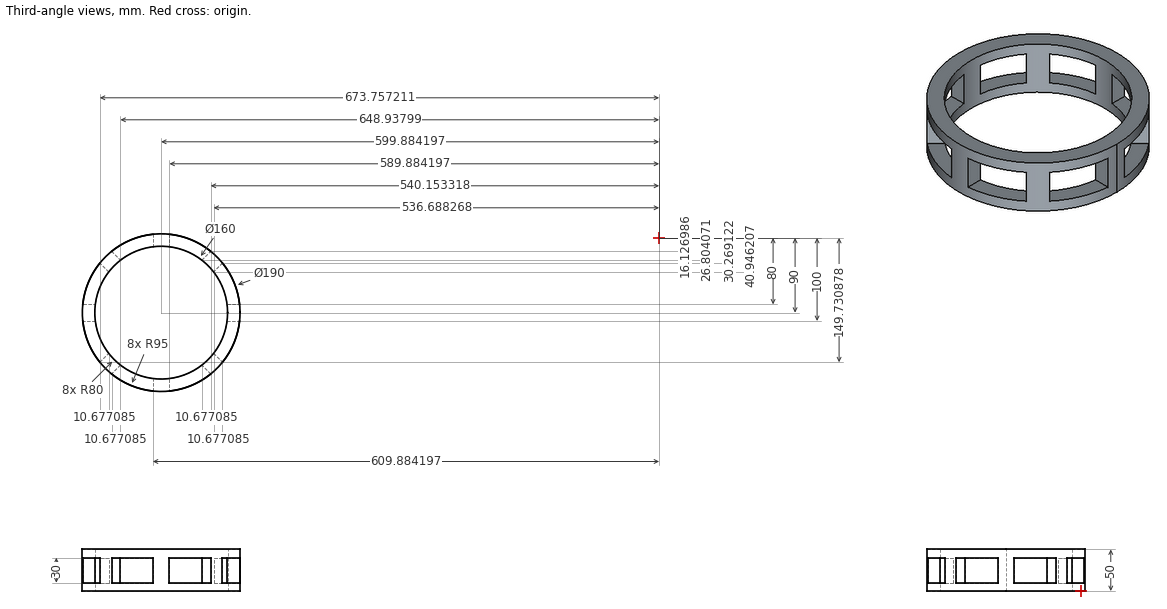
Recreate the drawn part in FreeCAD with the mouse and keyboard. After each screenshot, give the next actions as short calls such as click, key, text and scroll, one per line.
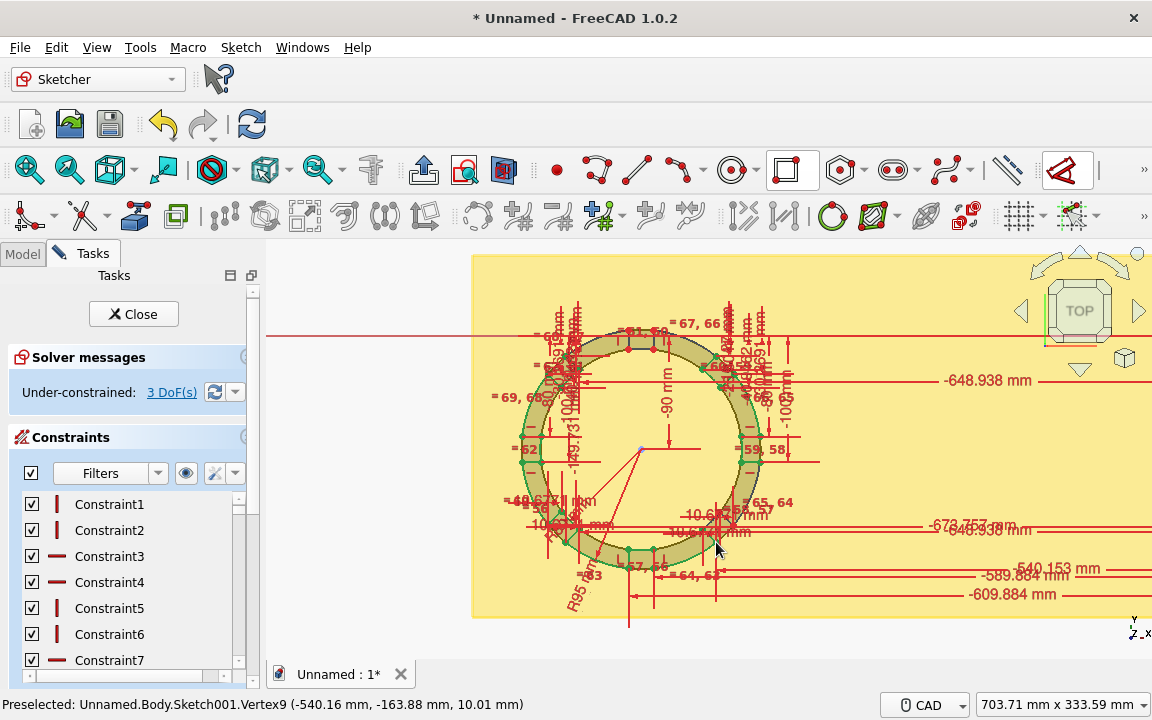
click(720, 512)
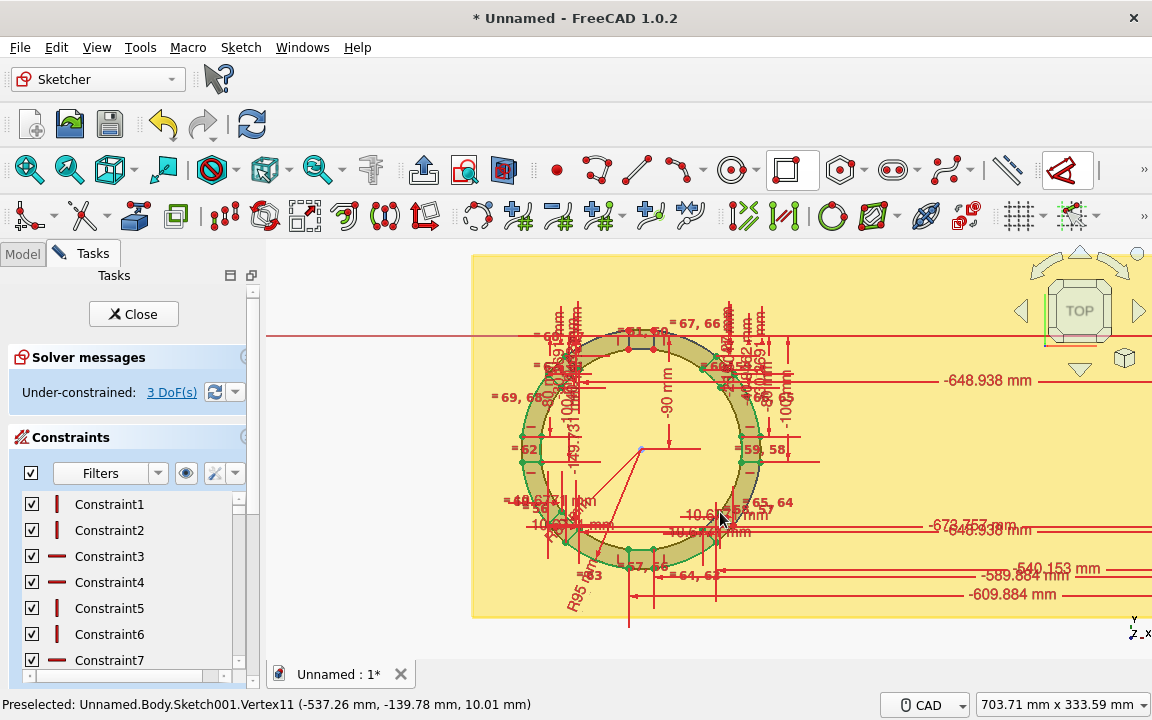
key(l)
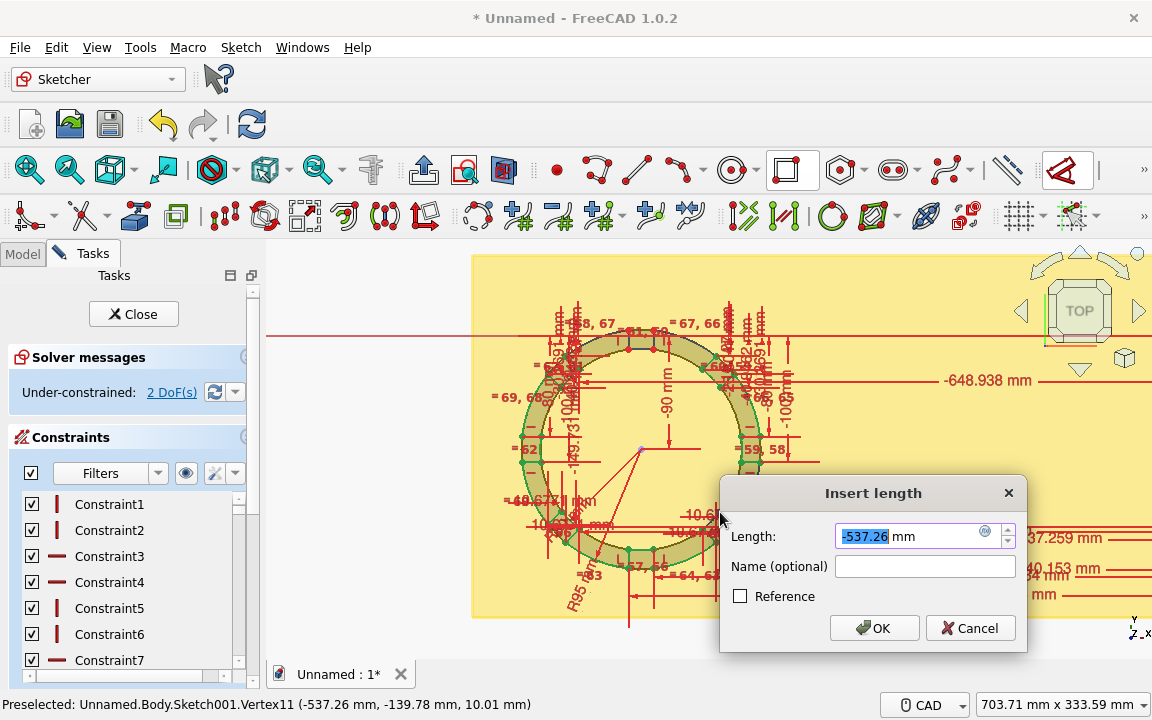
text(-536.688268)
key(Return)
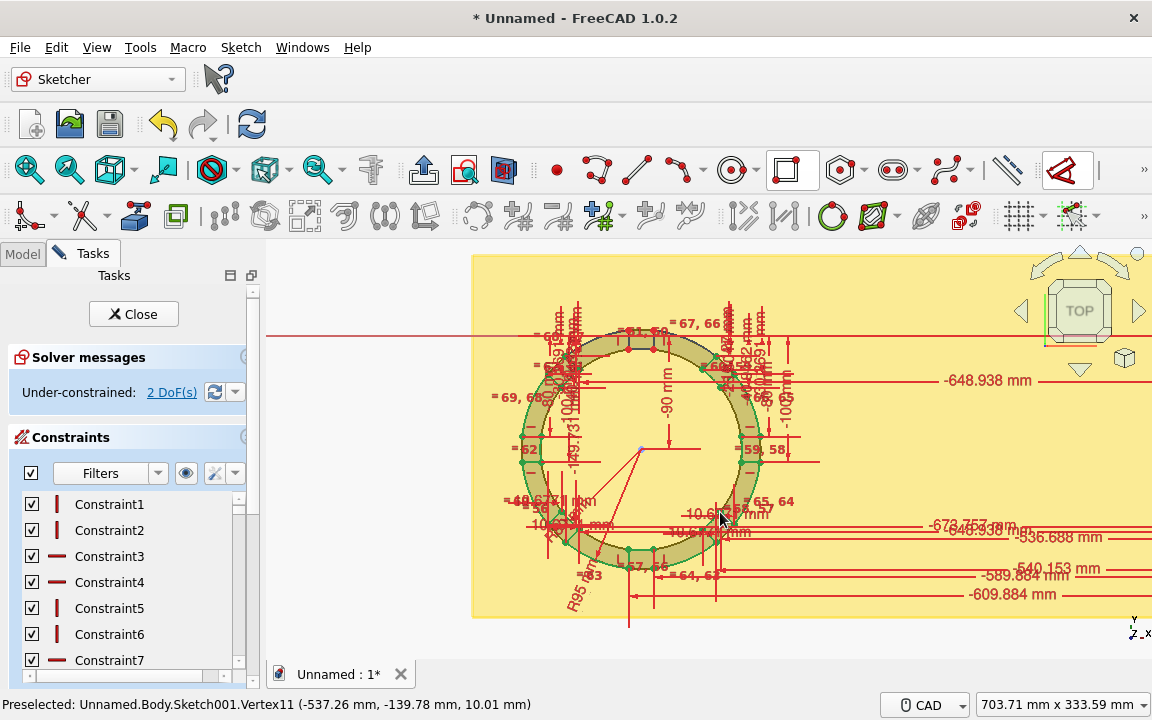
click(654, 331)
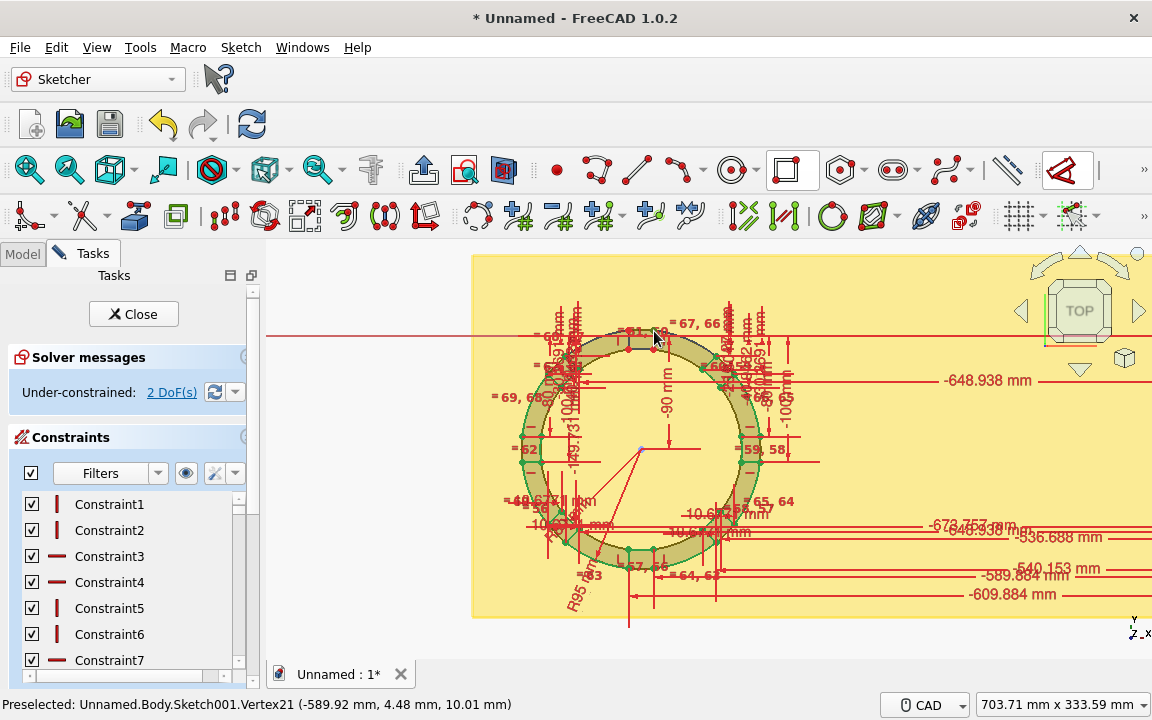
key(l)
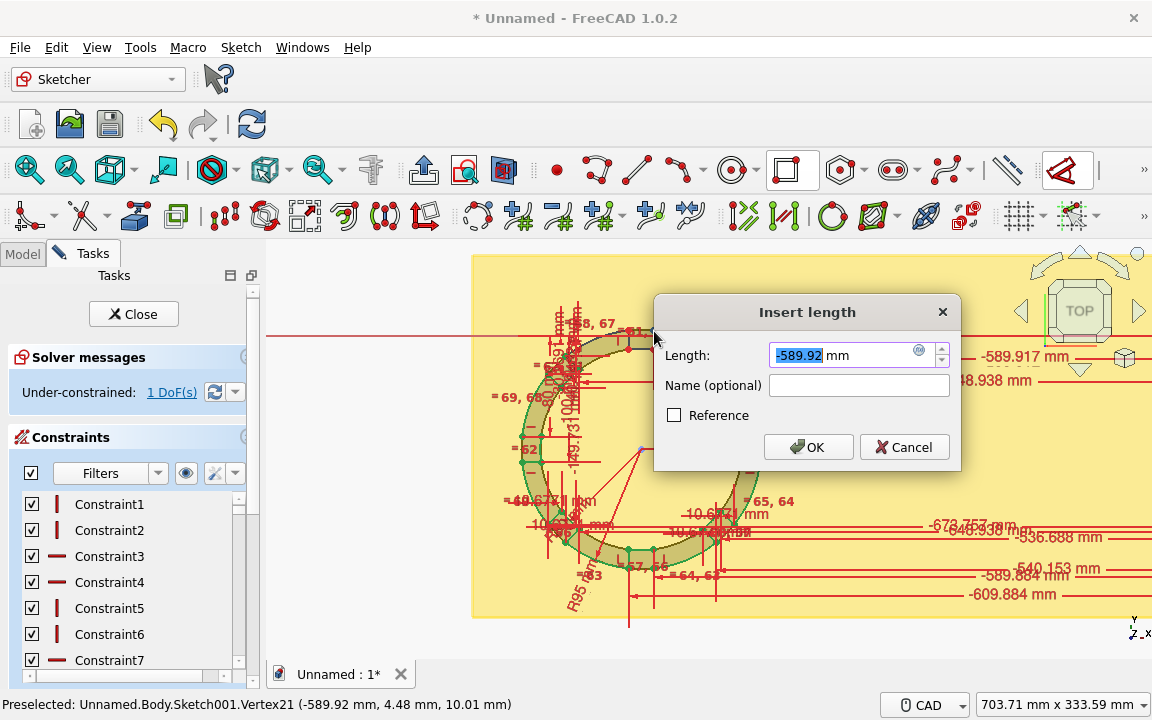
text(-589.884197)
key(Return)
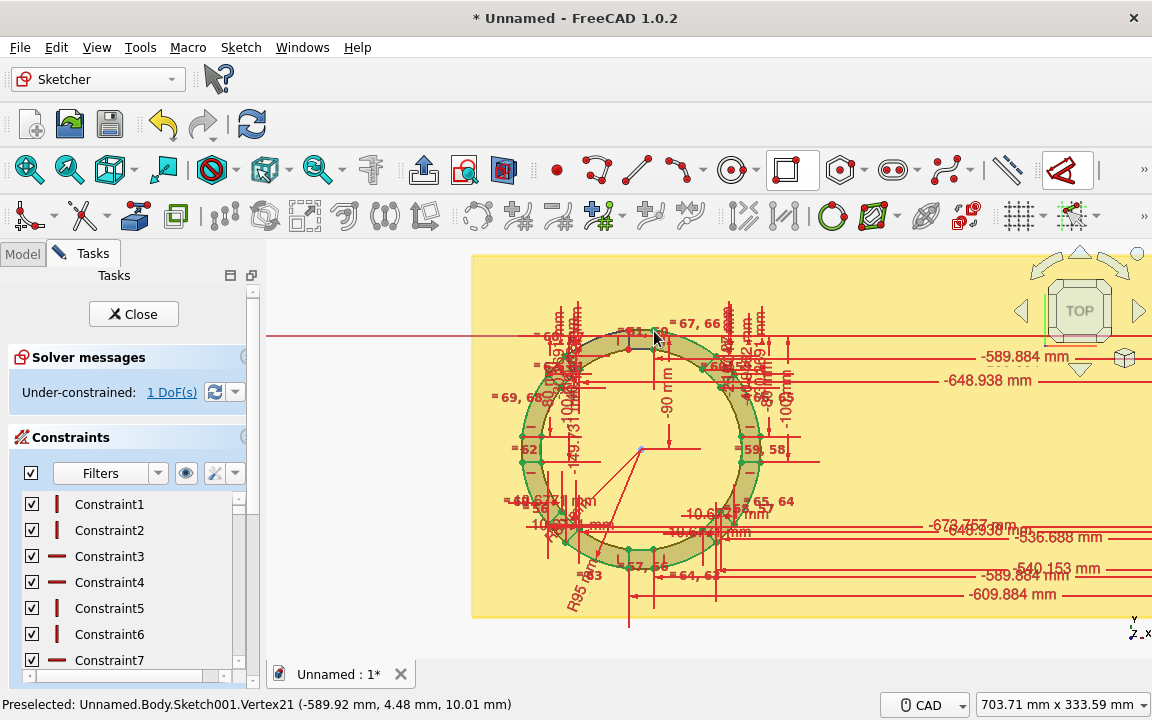
click(629, 350)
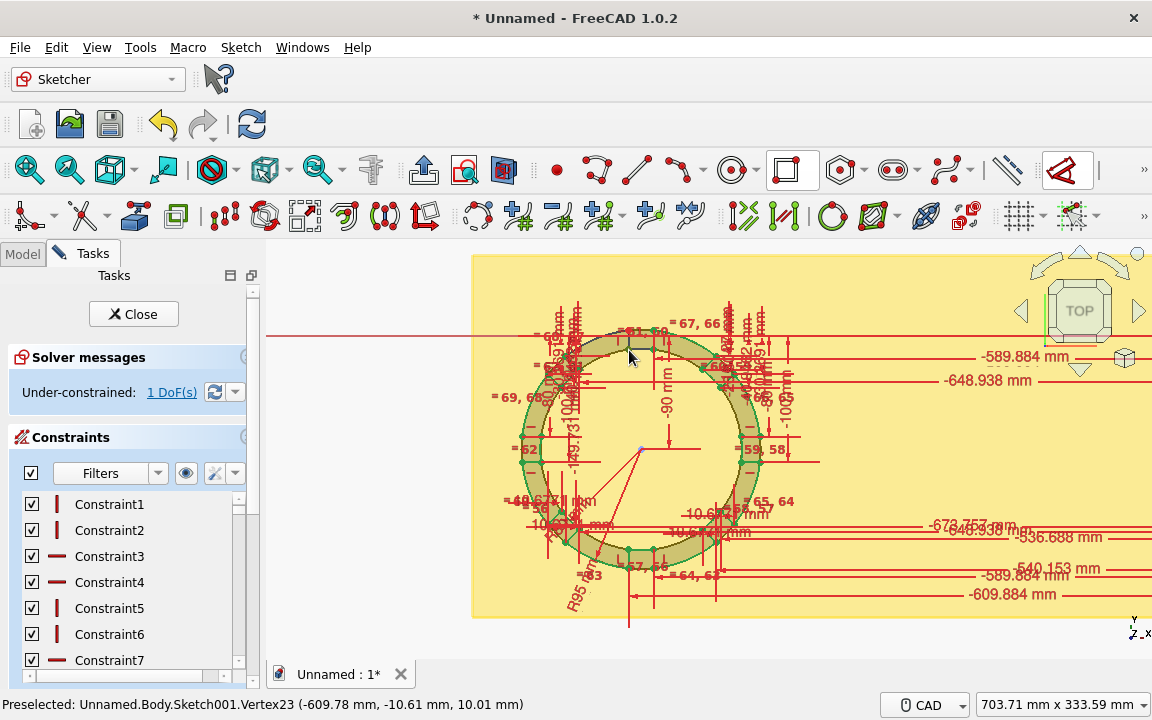
key(l)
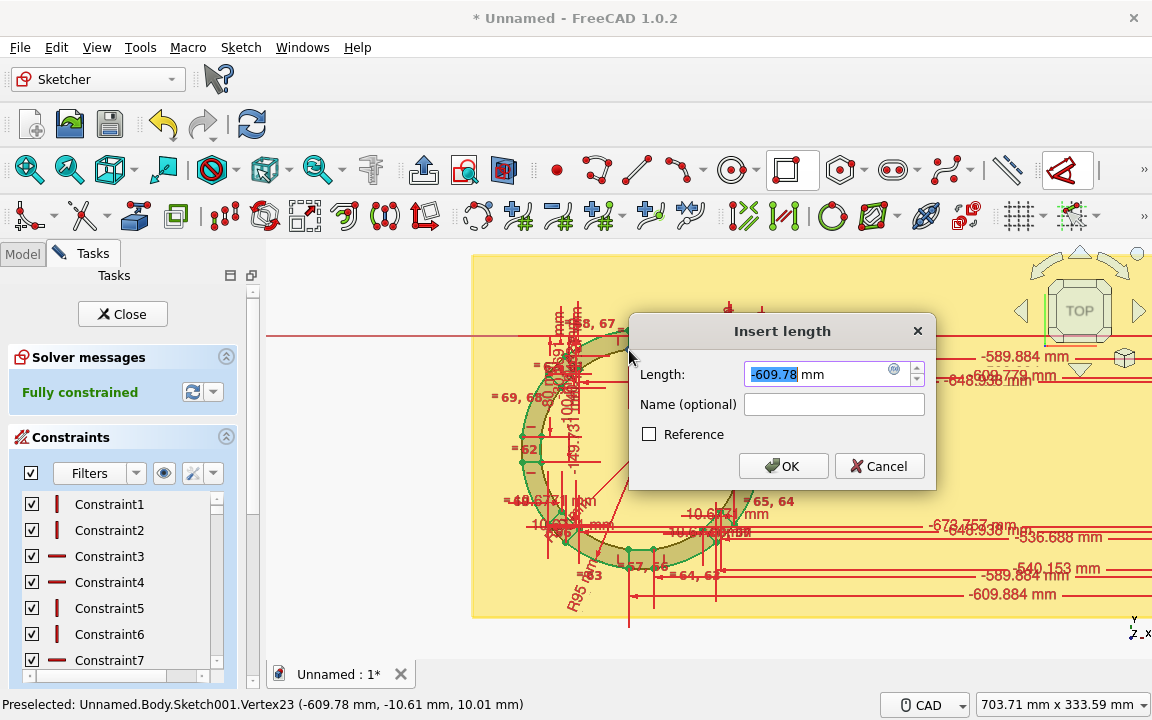
text(-609.884197)
key(Return)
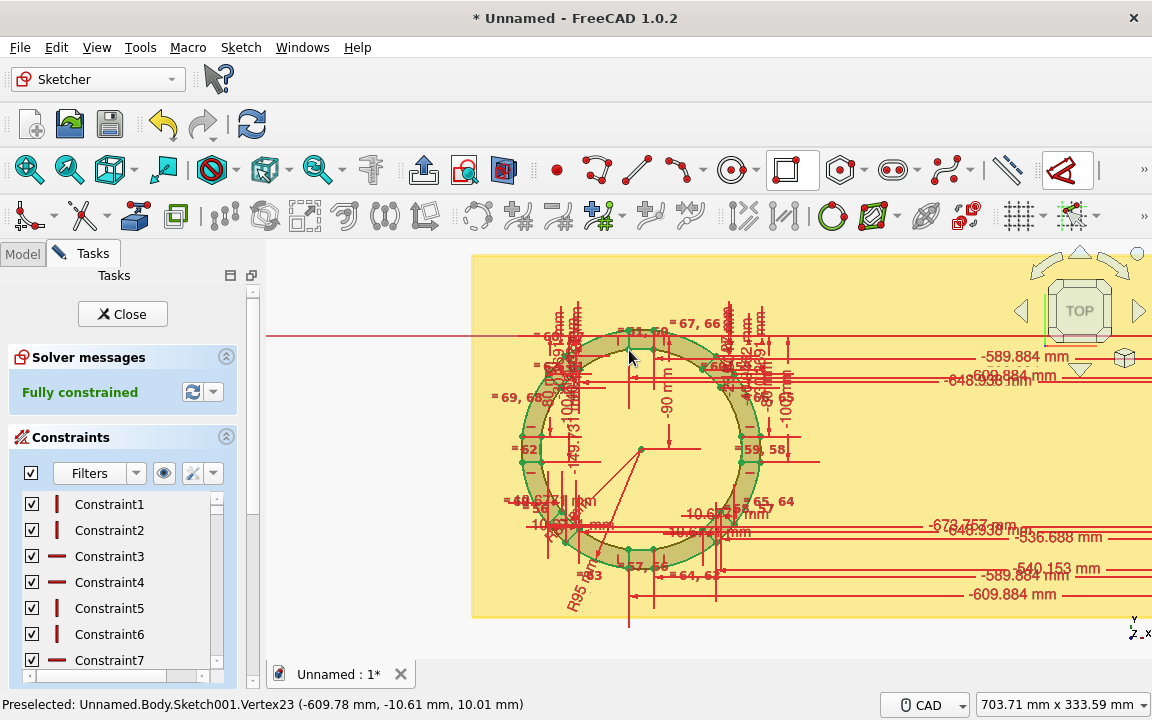
click(123, 314)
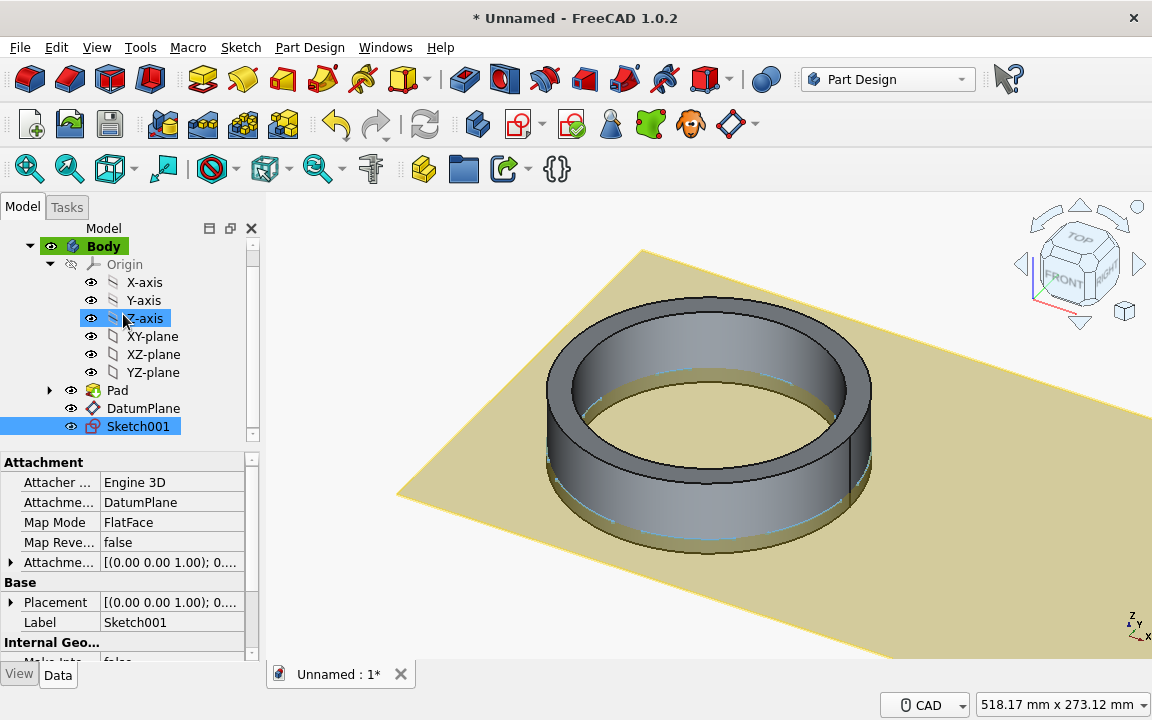
click(466, 80)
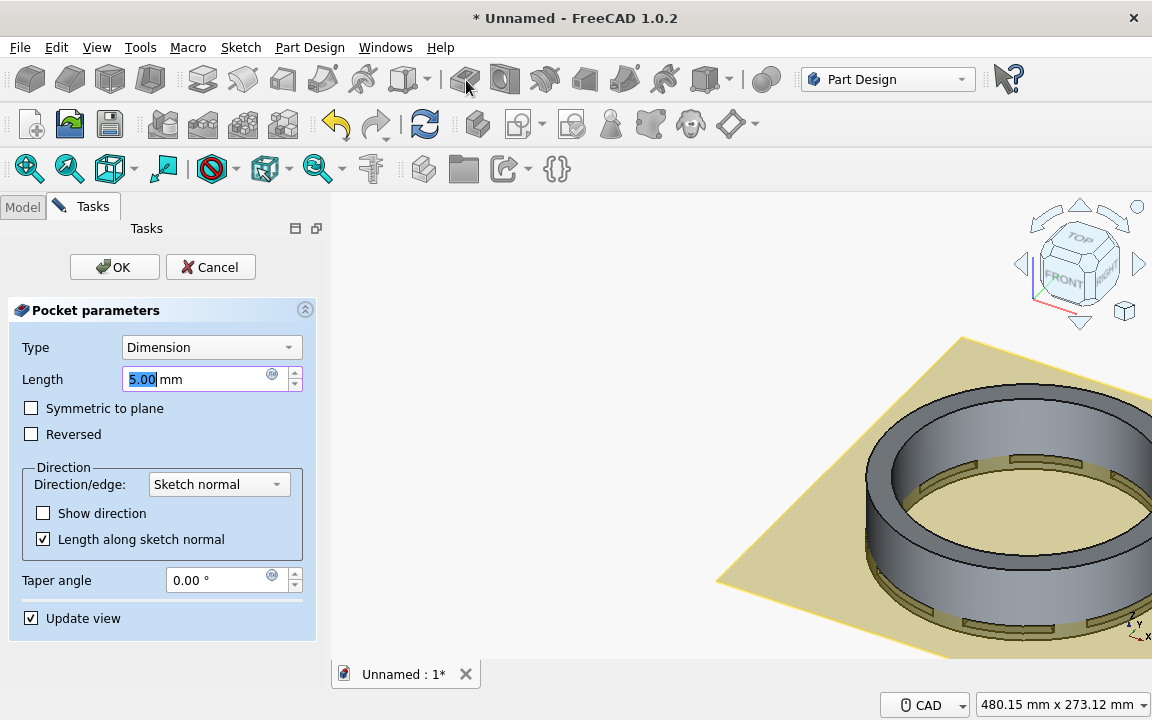
text(30)
key(Tab)